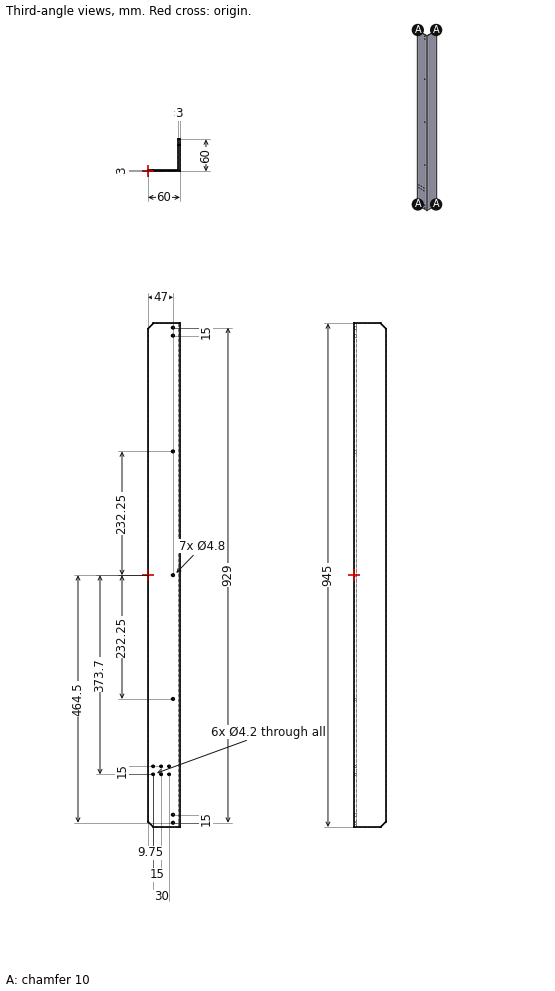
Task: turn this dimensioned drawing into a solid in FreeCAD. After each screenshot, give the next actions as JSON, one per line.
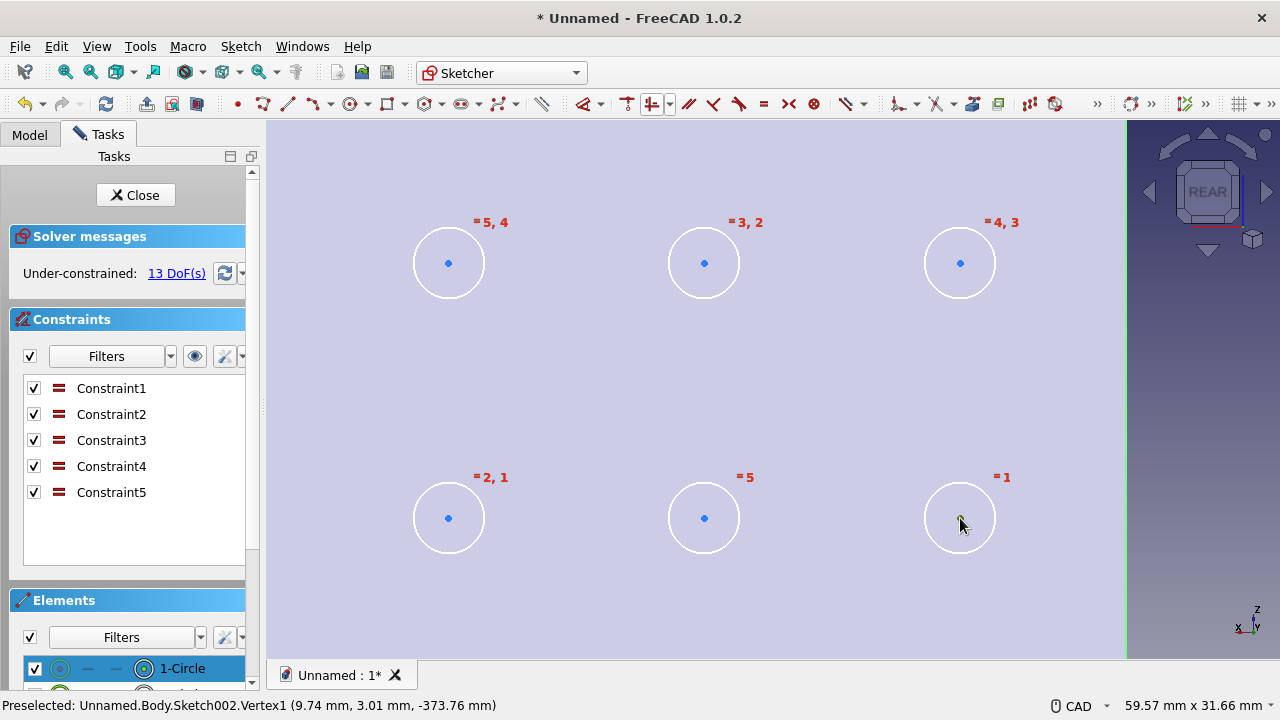
{"action": "left_click", "coordinate": [449, 518]}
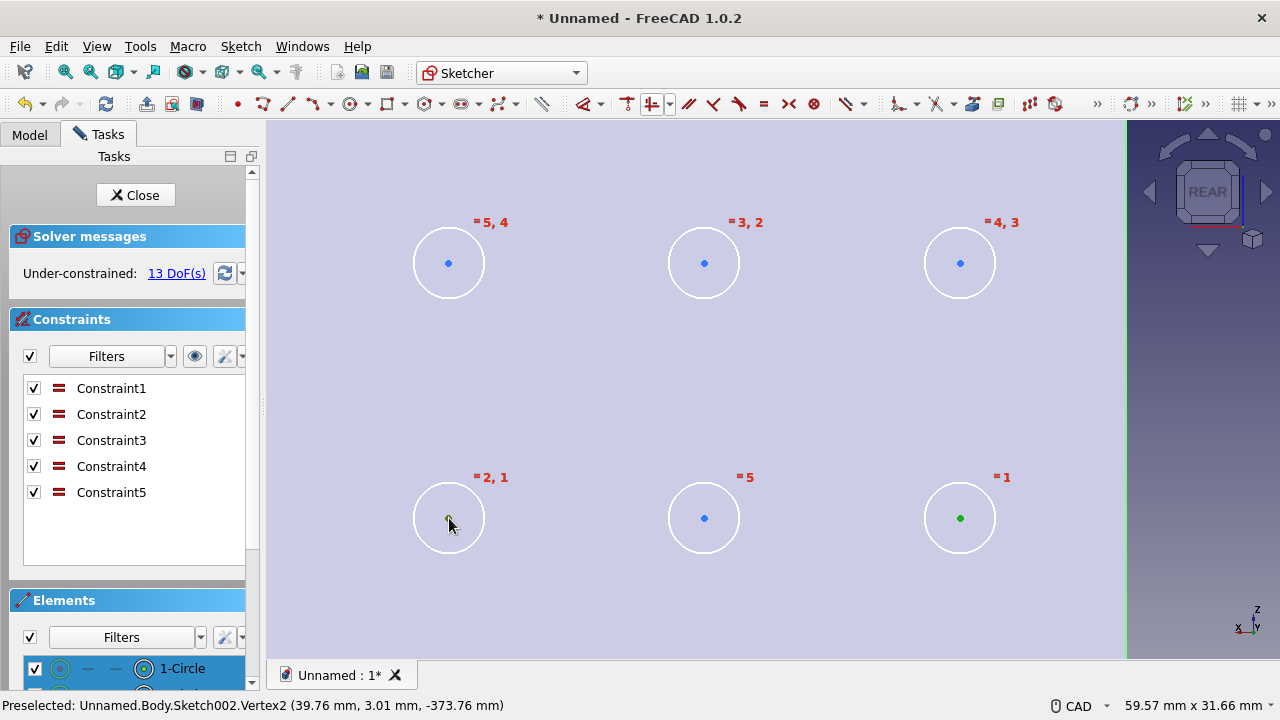
{"action": "left_click", "coordinate": [670, 104]}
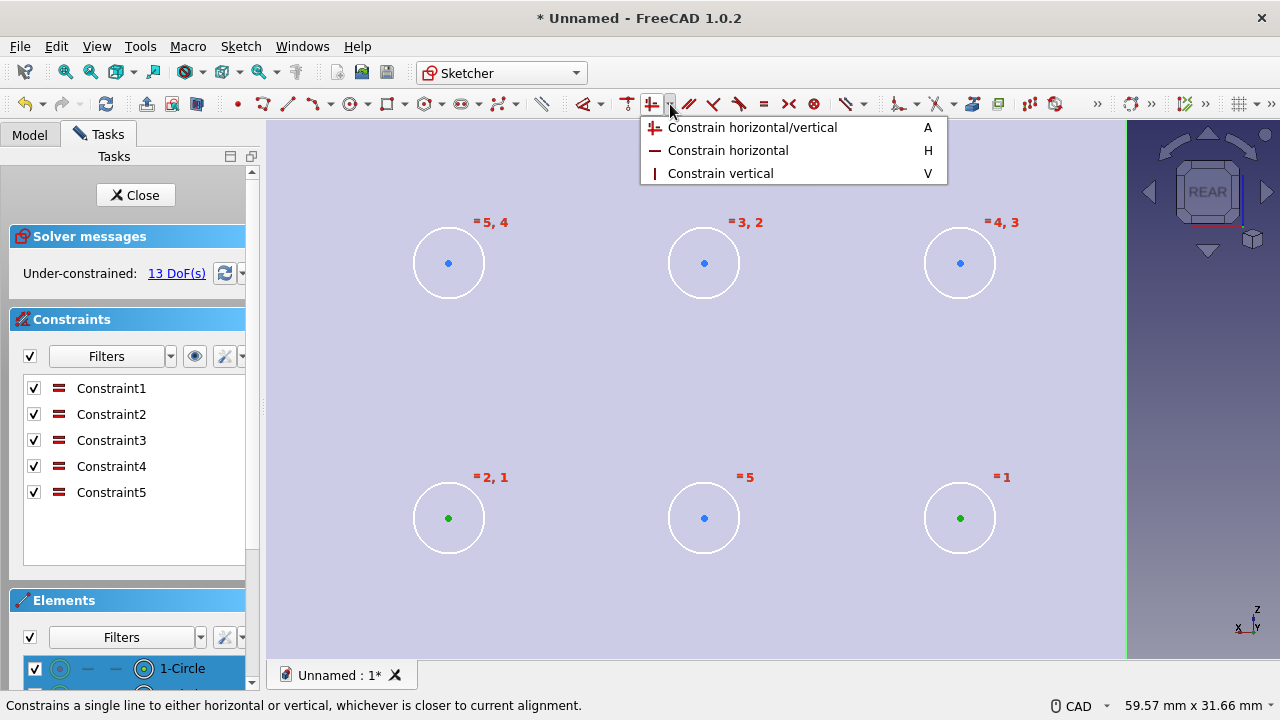
{"action": "left_click", "coordinate": [794, 150]}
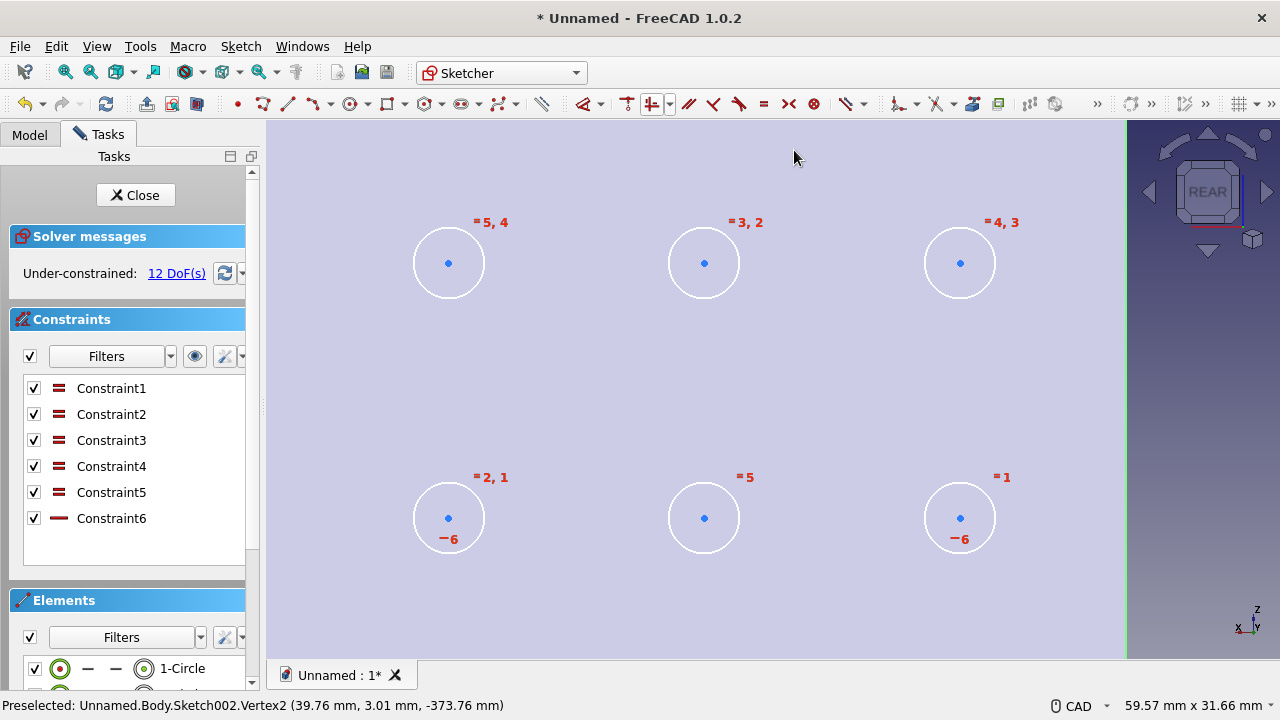
{"action": "left_click", "coordinate": [960, 518]}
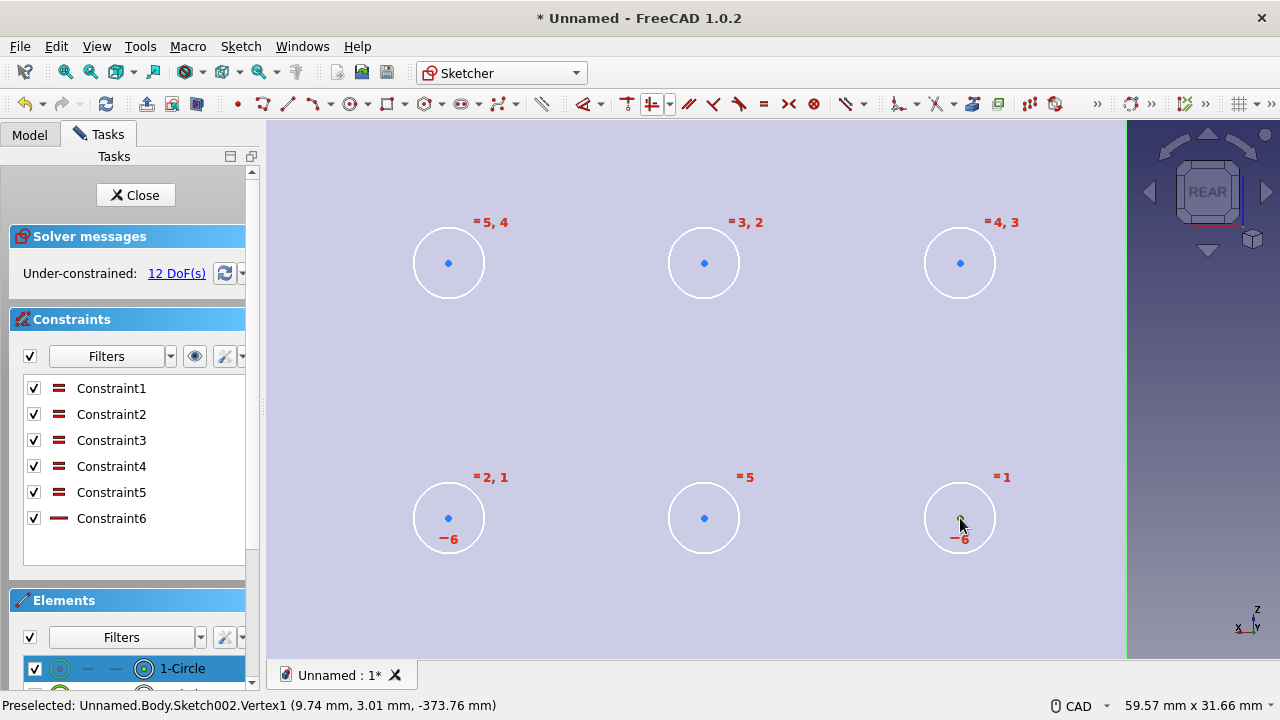
{"action": "left_click", "coordinate": [960, 263]}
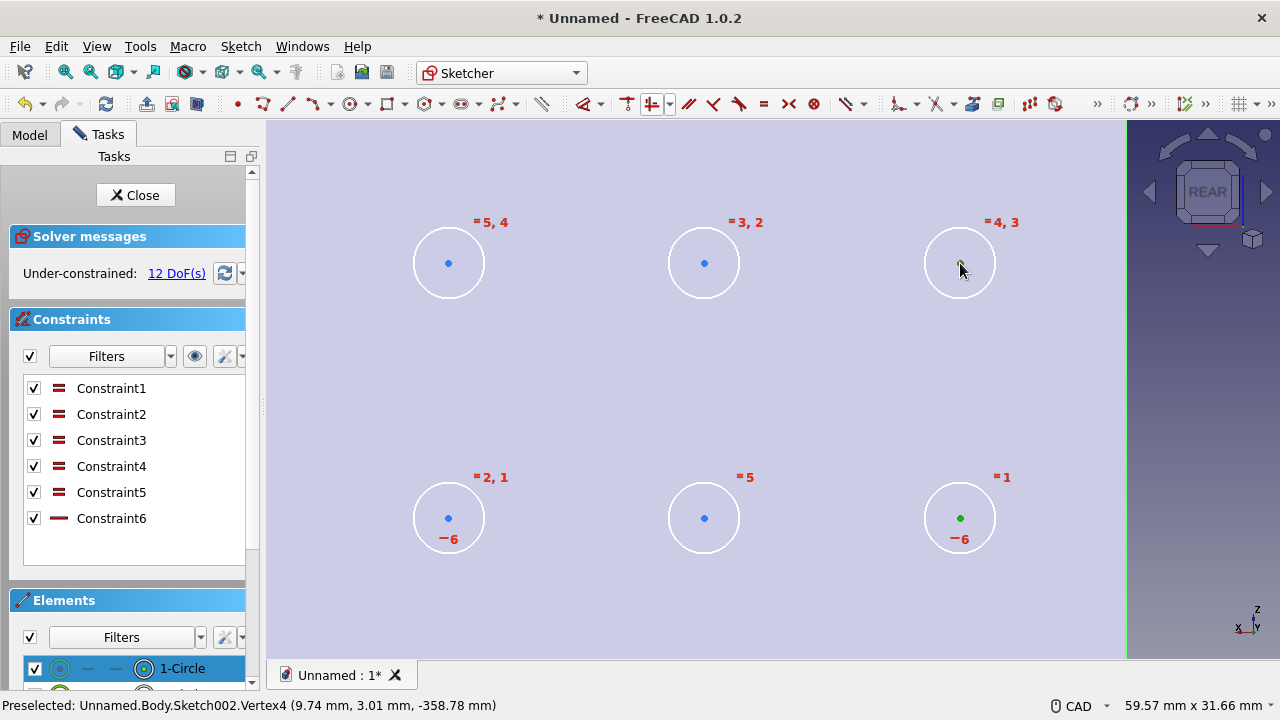
{"action": "key", "text": "v"}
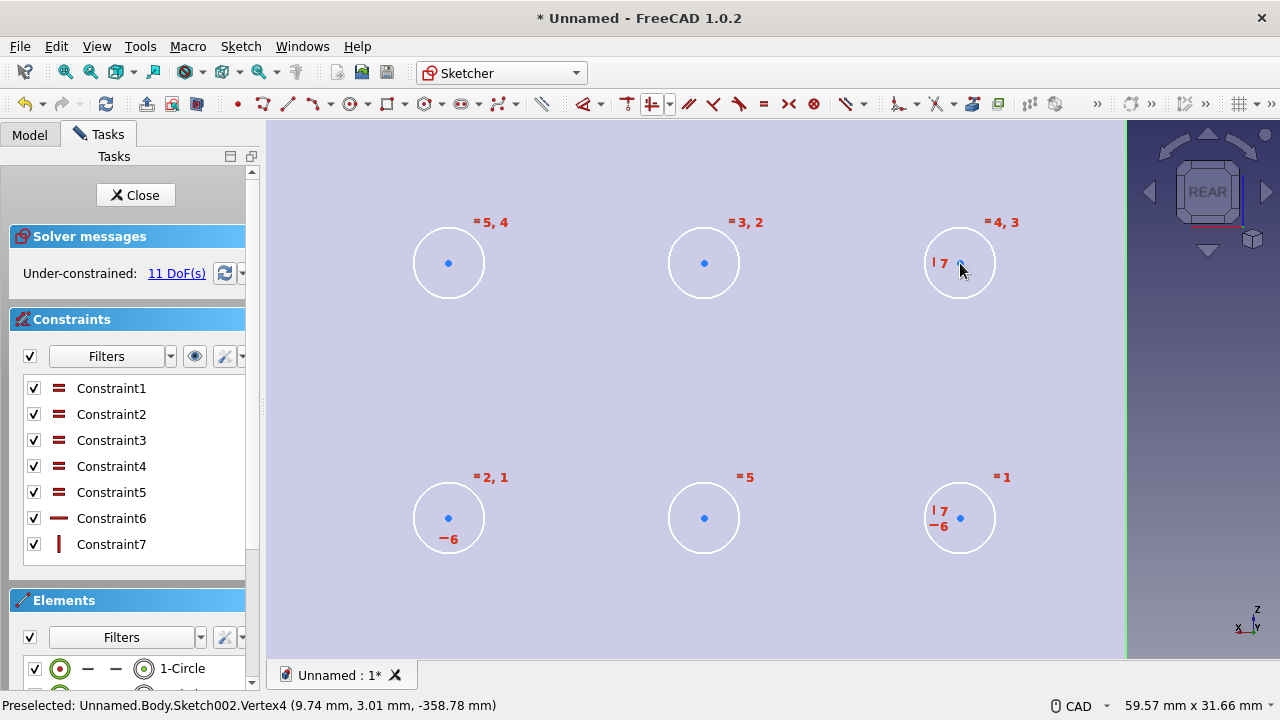
{"action": "left_click", "coordinate": [704, 263]}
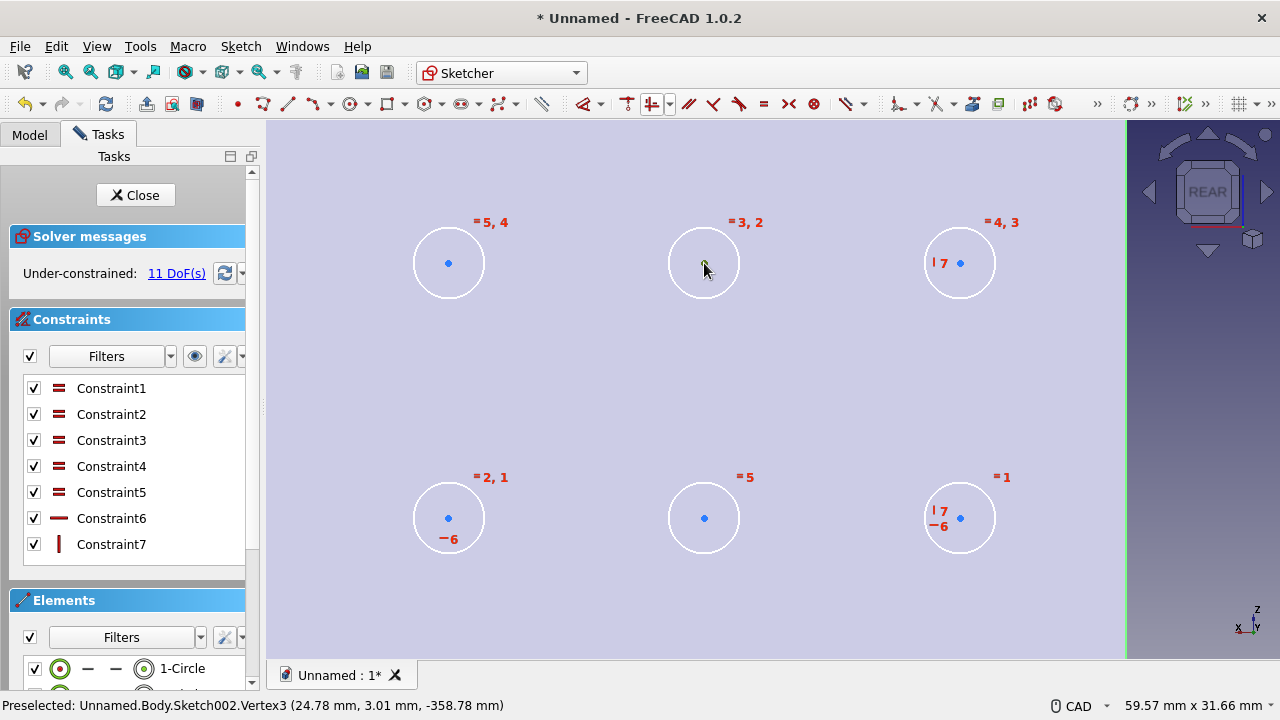
{"action": "left_click", "coordinate": [960, 263]}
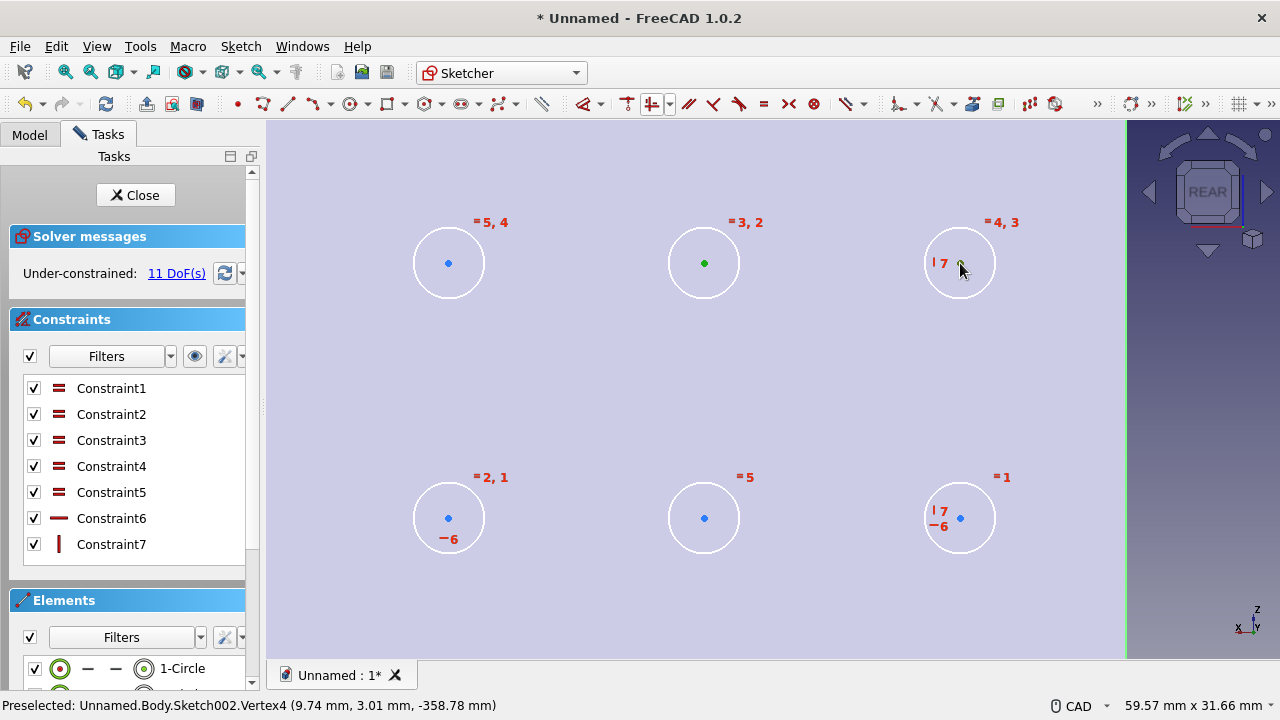
{"action": "left_click", "coordinate": [670, 104]}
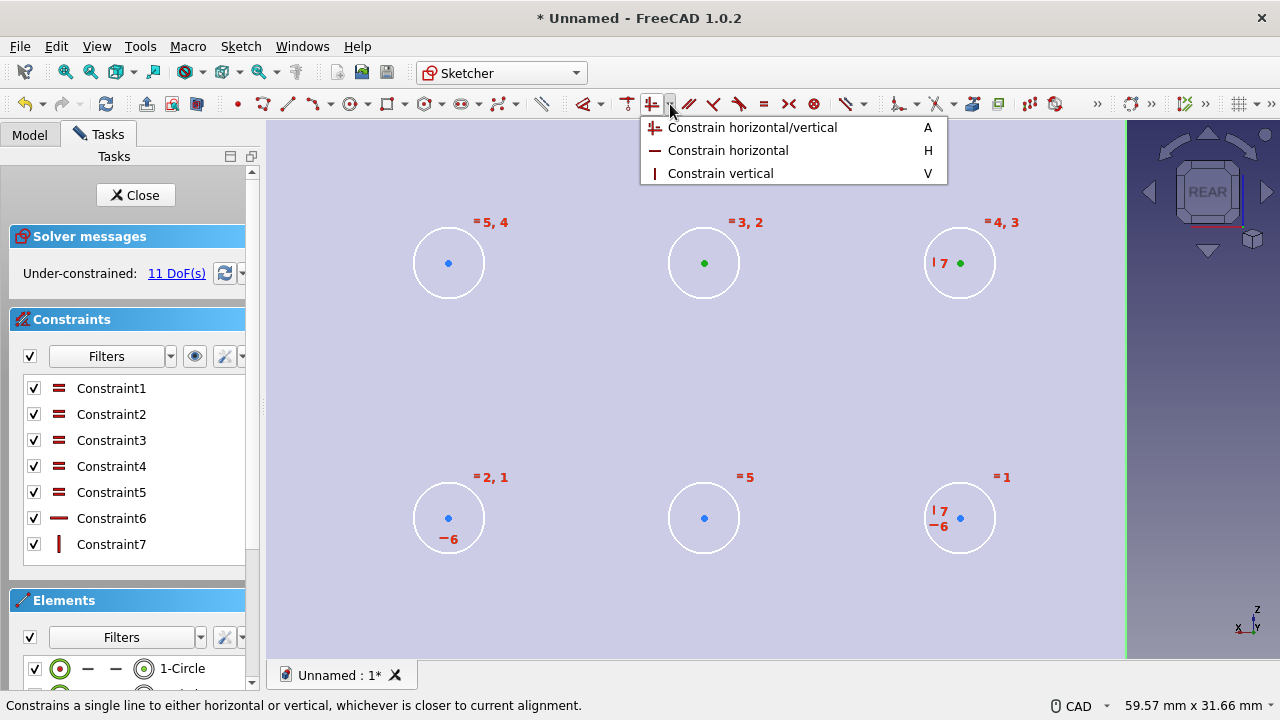
{"action": "left_click", "coordinate": [794, 150]}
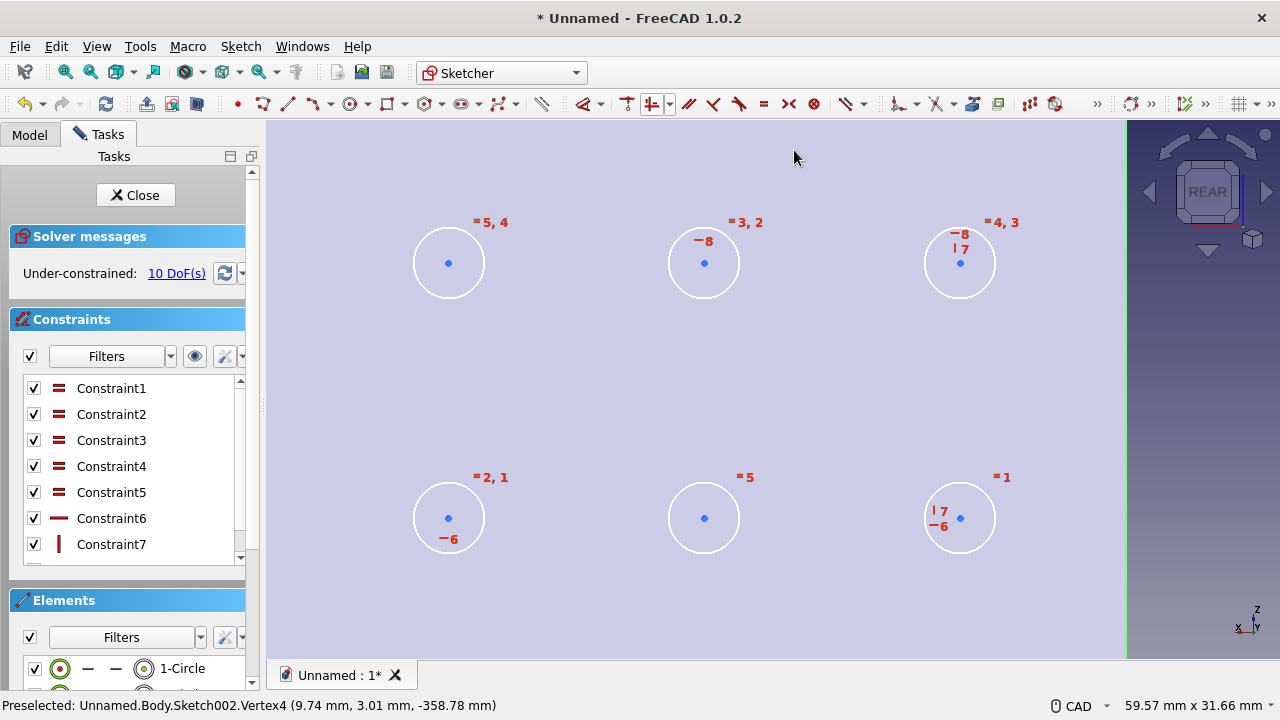
{"action": "left_click", "coordinate": [449, 518]}